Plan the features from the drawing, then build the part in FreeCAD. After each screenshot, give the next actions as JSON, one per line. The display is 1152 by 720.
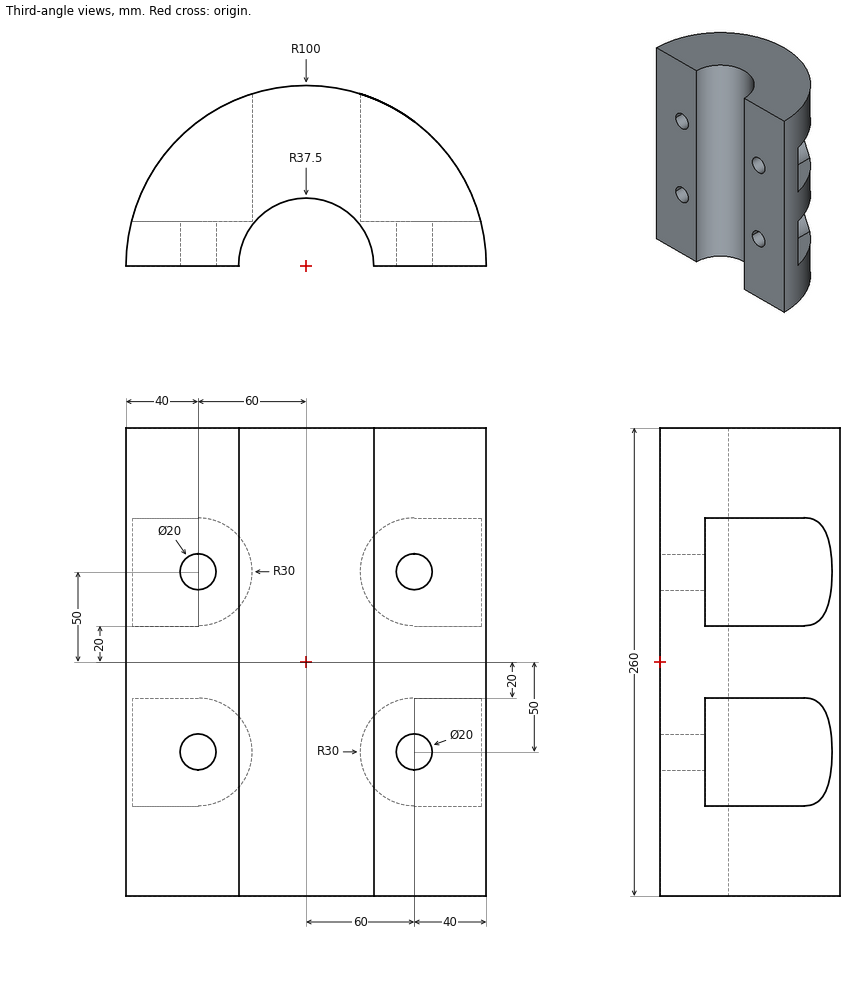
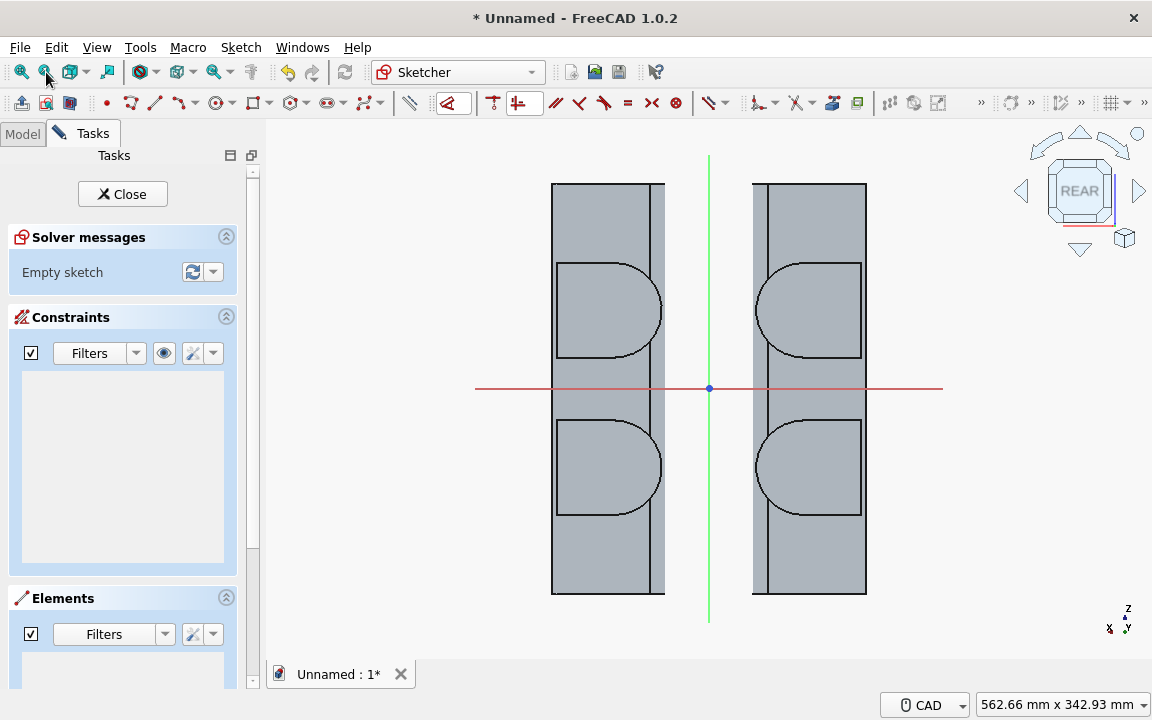
{"action": "scroll", "coordinate": [820, 302], "scroll_direction": "up", "scroll_amount": 12}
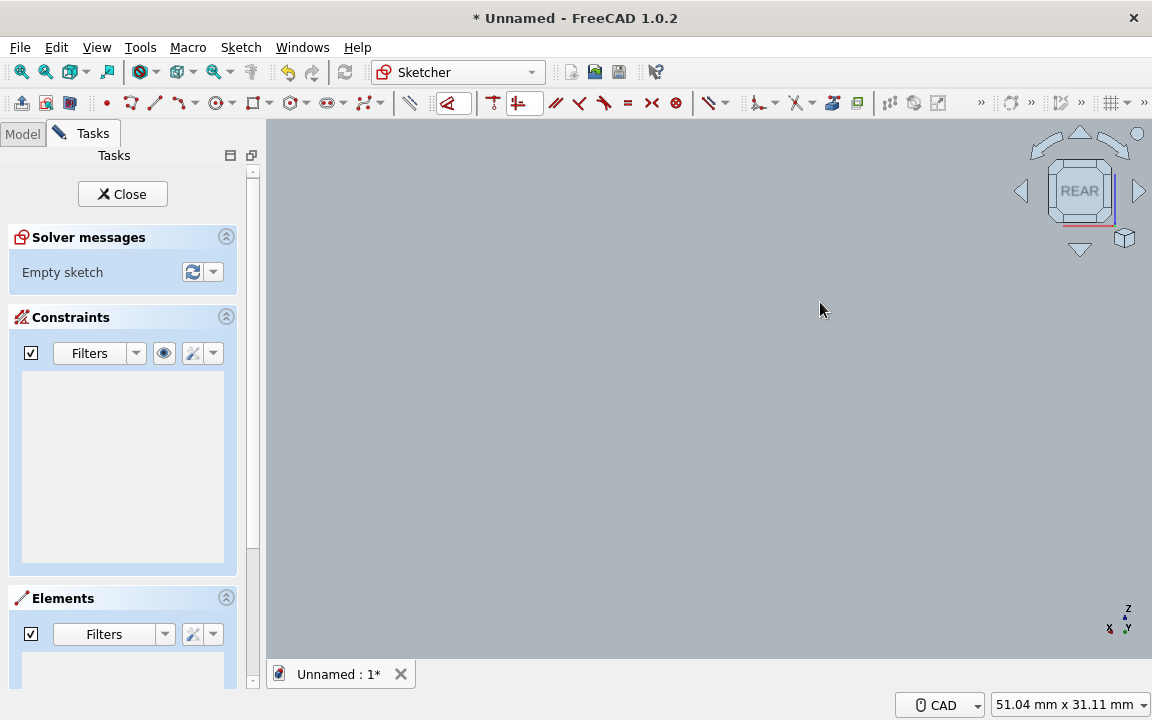
{"action": "key", "text": "g c"}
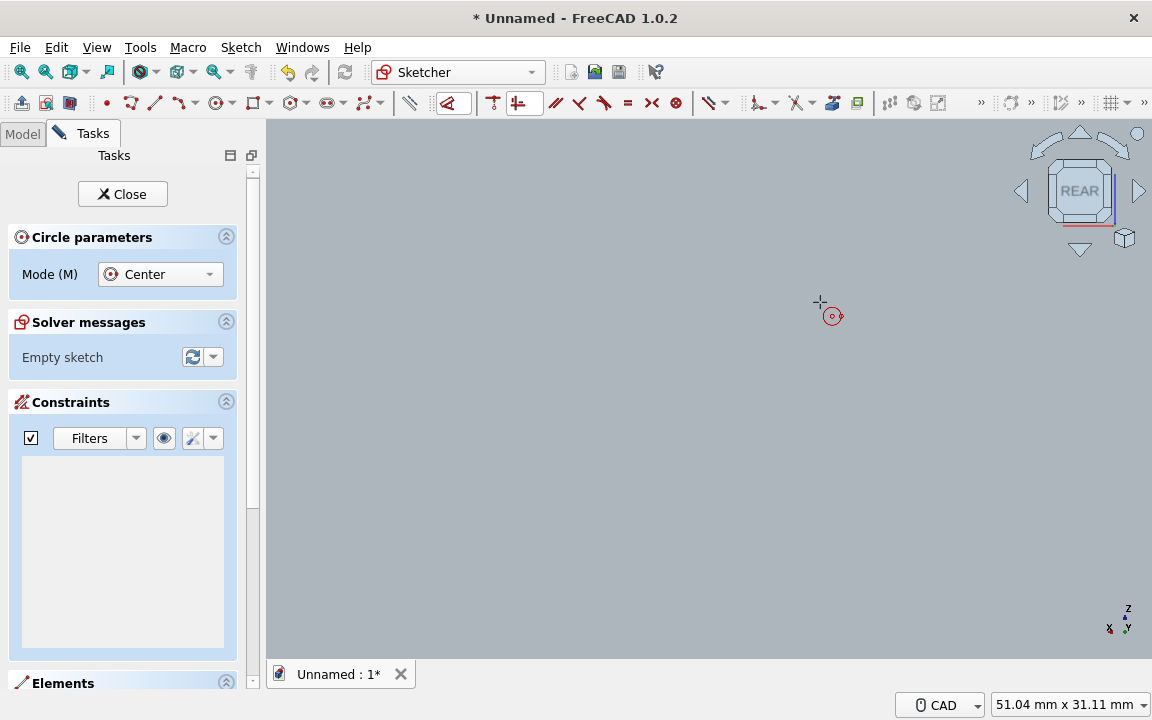
{"action": "left_click", "coordinate": [632, 390]}
{"action": "left_click", "coordinate": [754, 267]}
{"action": "key", "text": "Escape"}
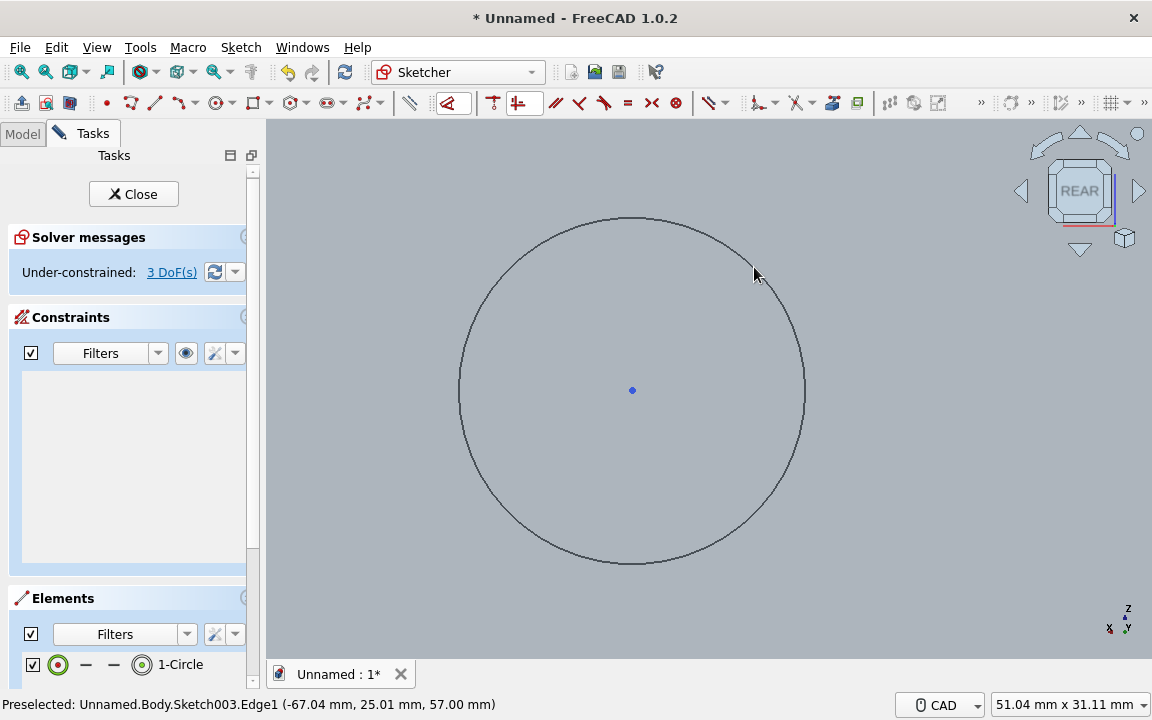
{"action": "left_click", "coordinate": [754, 268]}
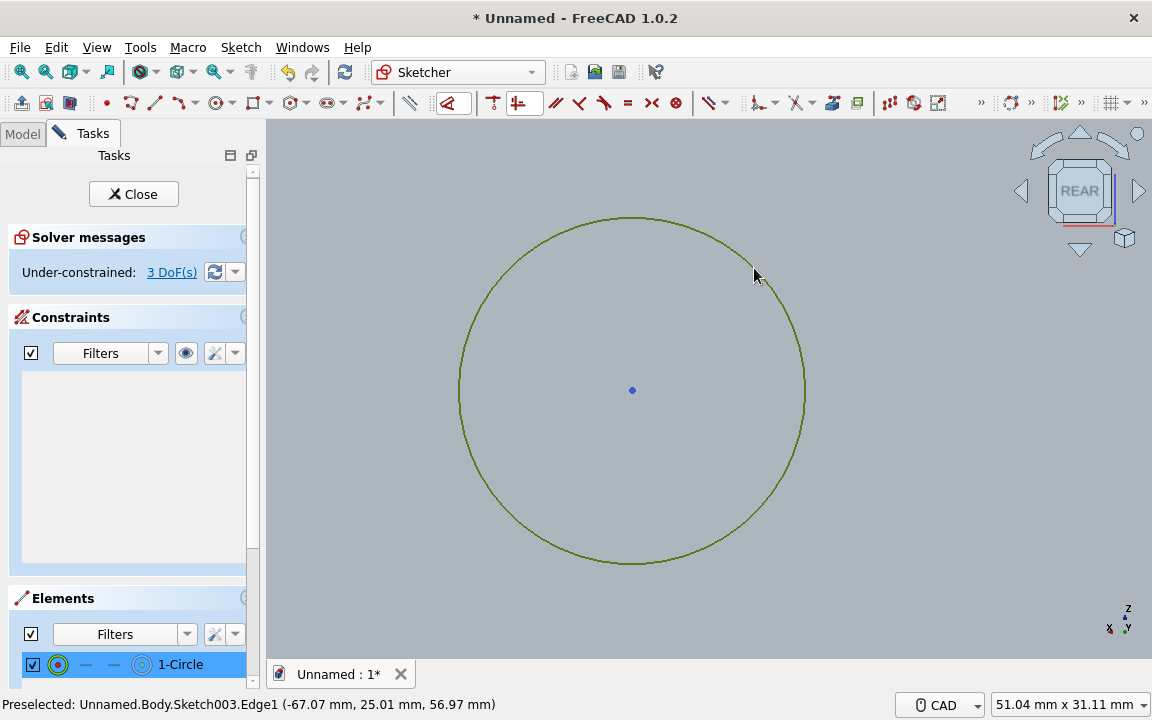
{"action": "key", "text": "k o"}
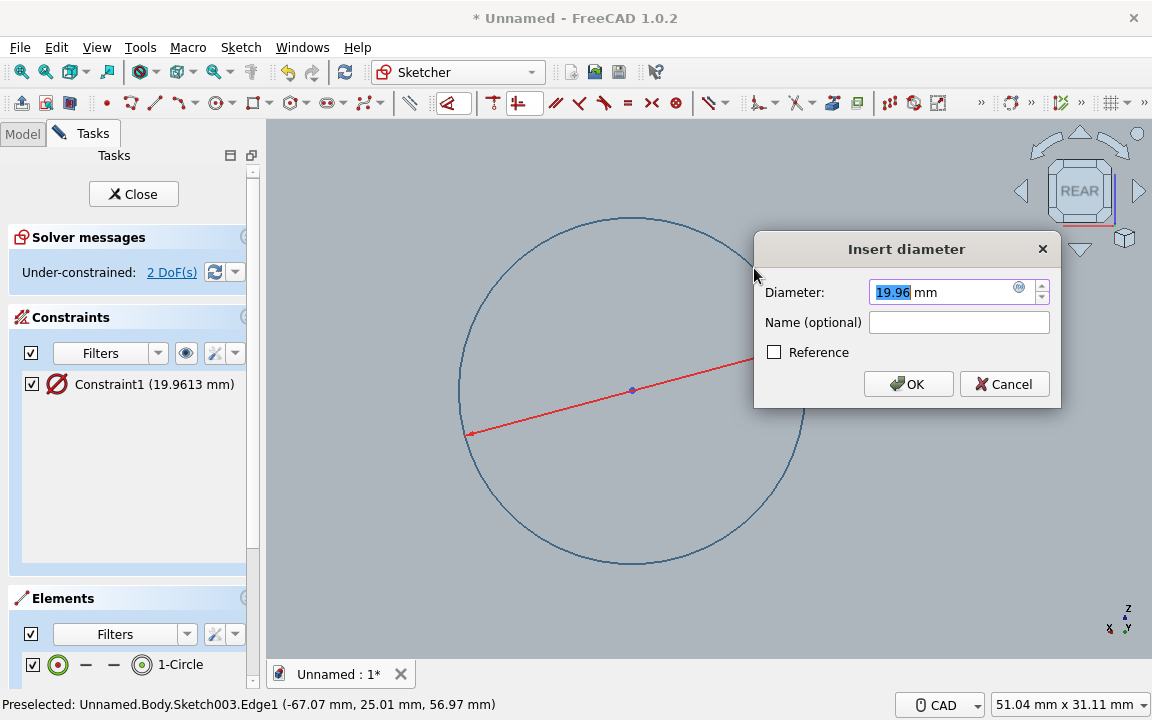
{"action": "type", "text": "20"}
{"action": "key", "text": "Return"}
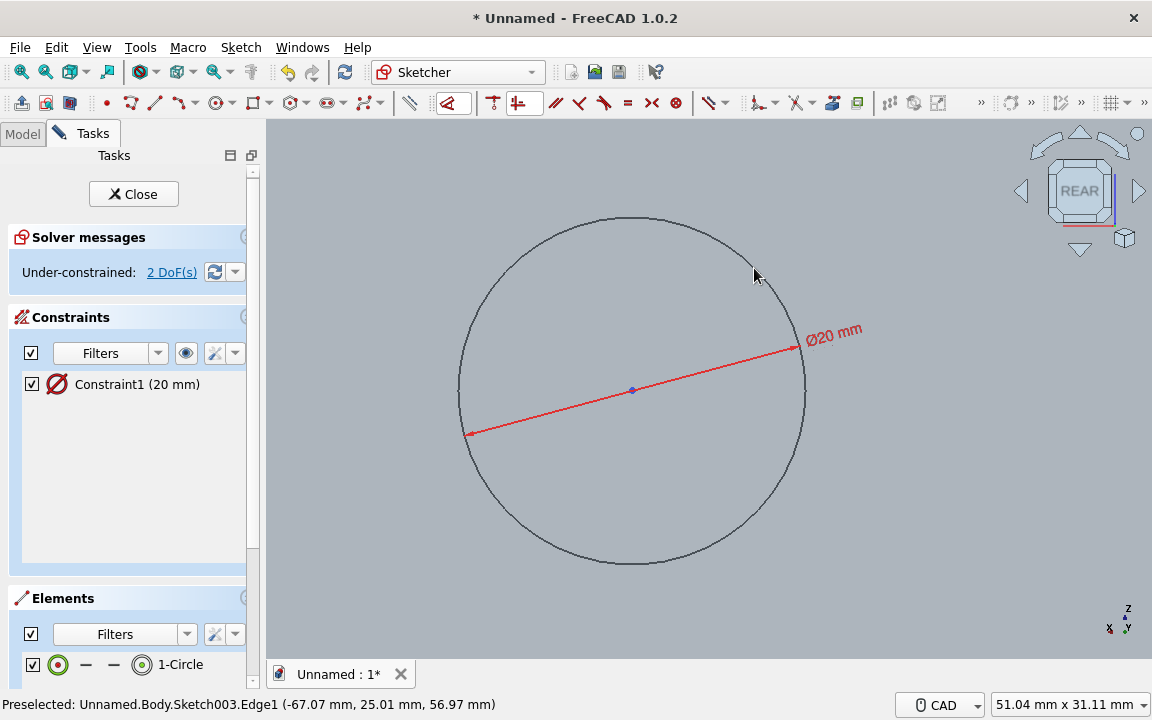
{"action": "left_click", "coordinate": [632, 391]}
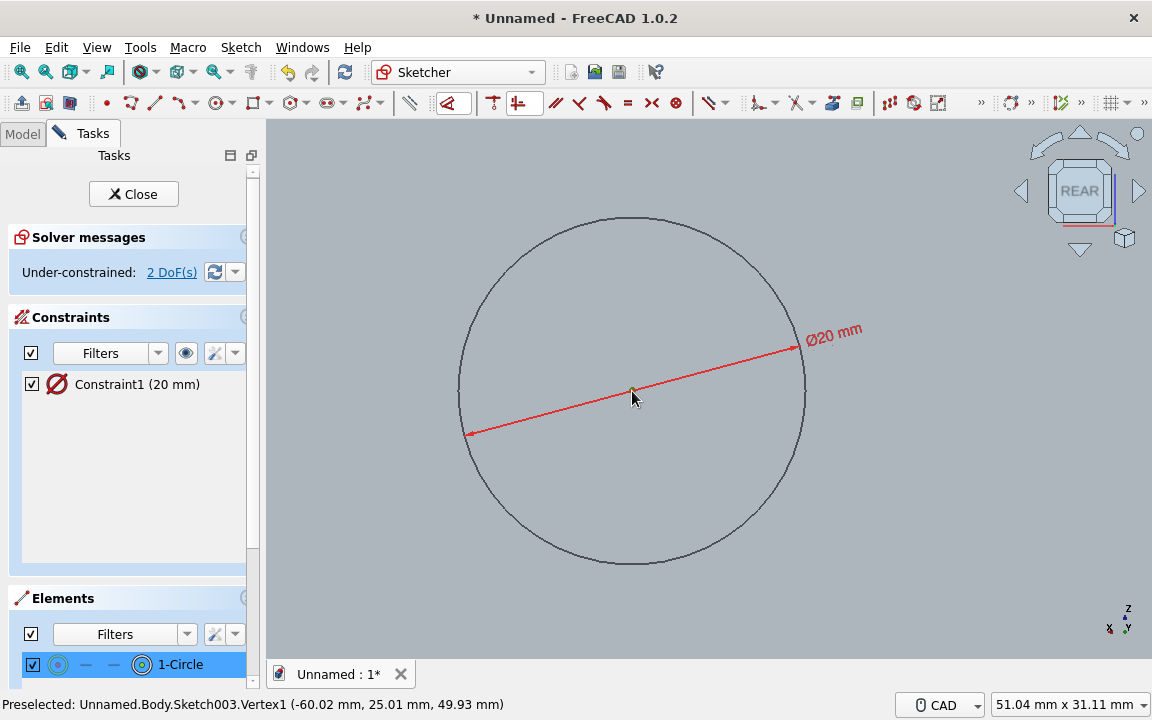
{"action": "key", "text": "l"}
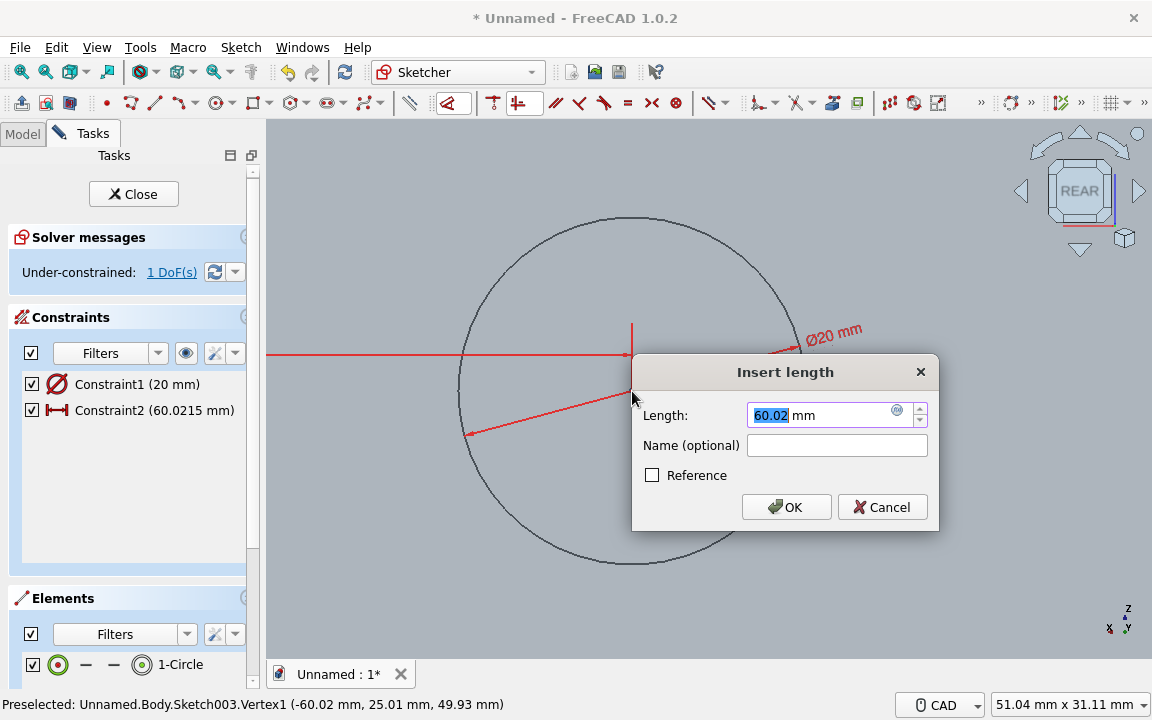
{"action": "type", "text": "60"}
{"action": "key", "text": "Return"}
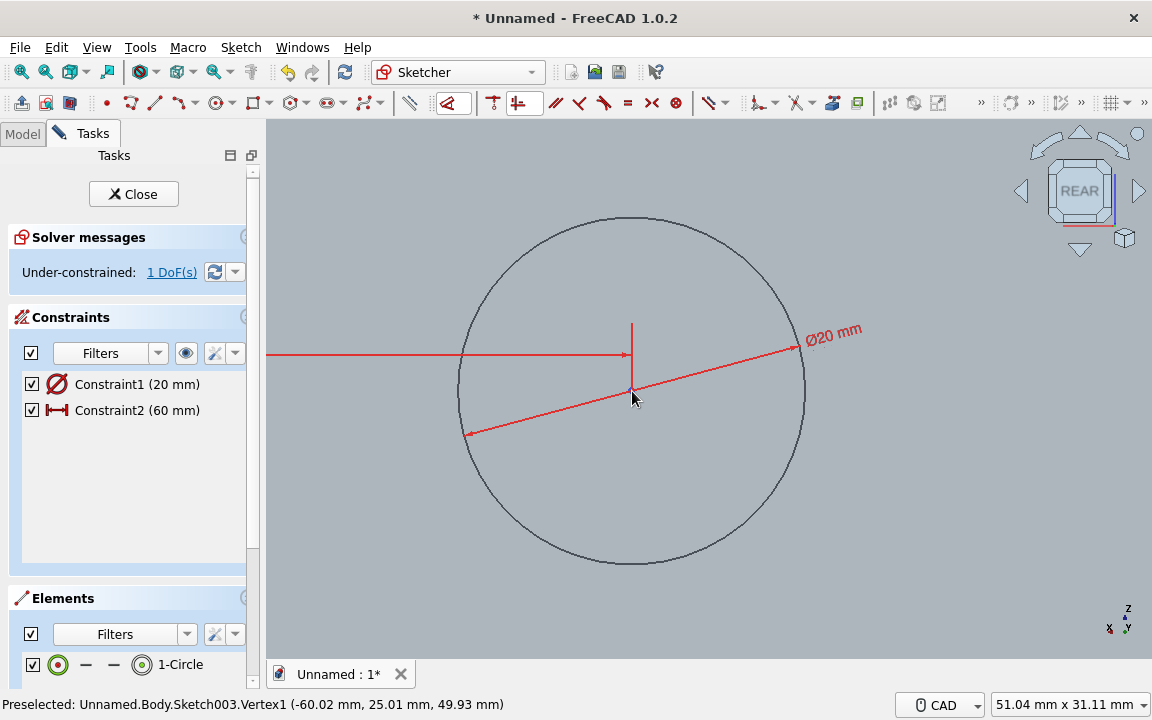
{"action": "left_click", "coordinate": [632, 391]}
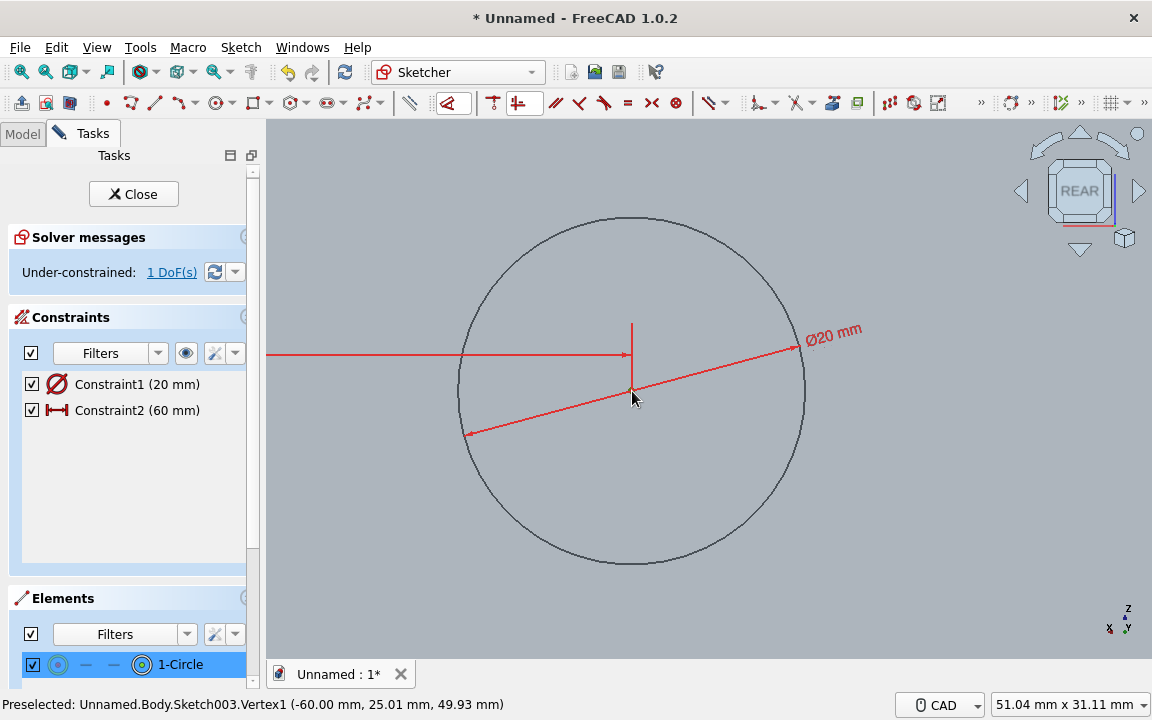
{"action": "key", "text": "i"}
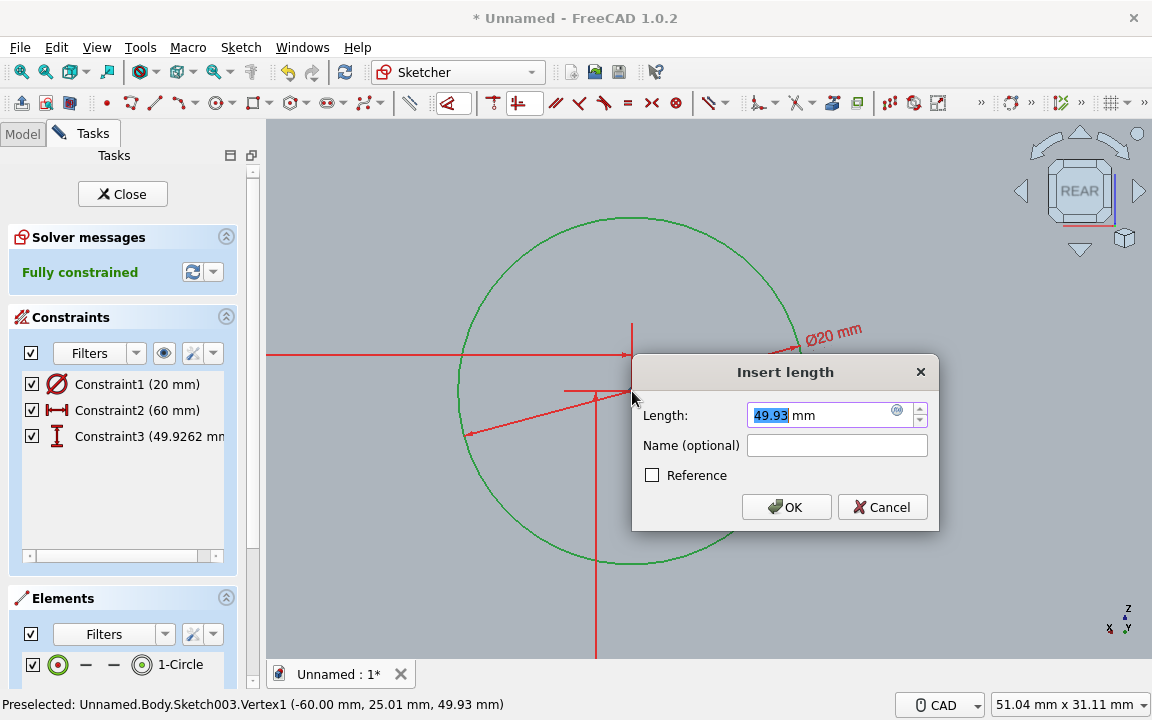
{"action": "type", "text": "50"}
{"action": "key", "text": "Return"}